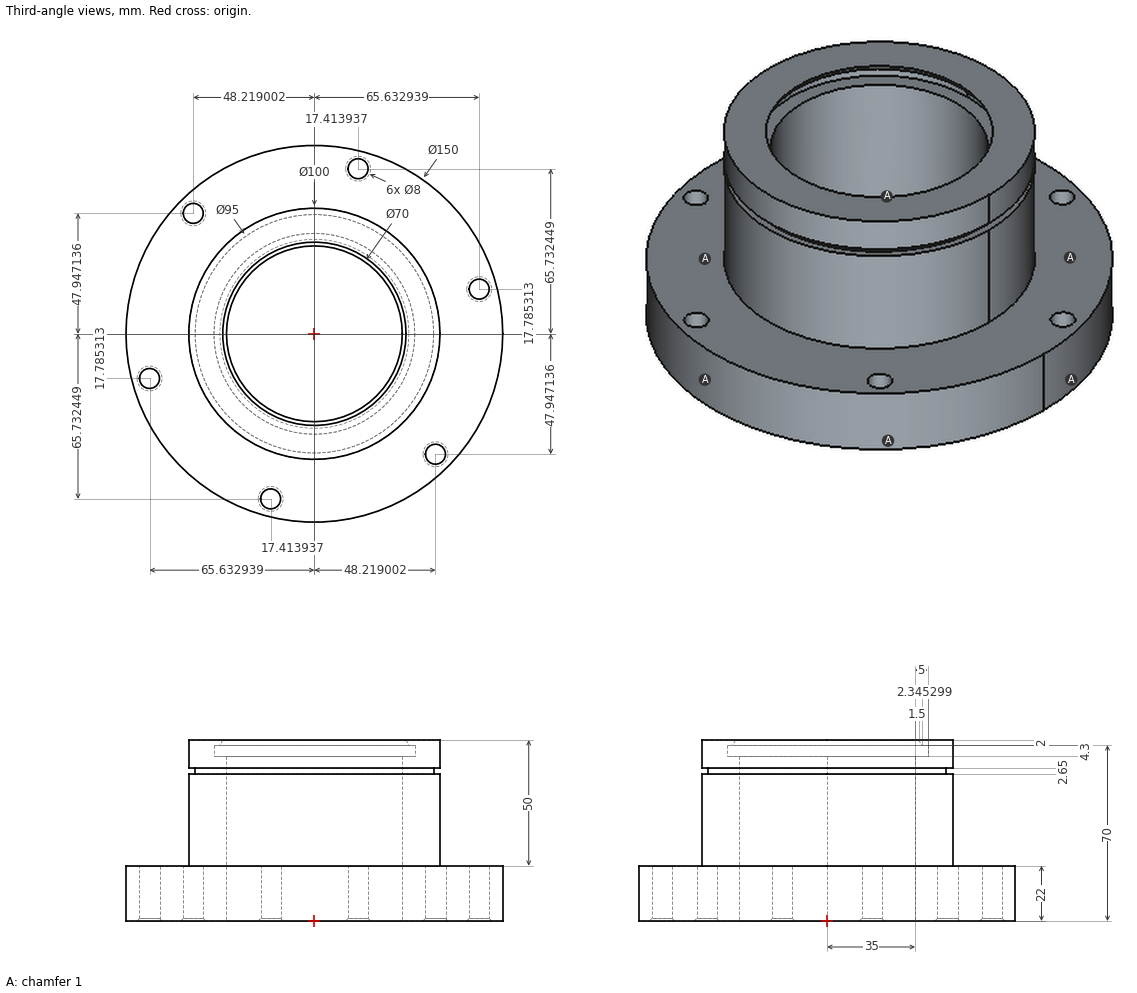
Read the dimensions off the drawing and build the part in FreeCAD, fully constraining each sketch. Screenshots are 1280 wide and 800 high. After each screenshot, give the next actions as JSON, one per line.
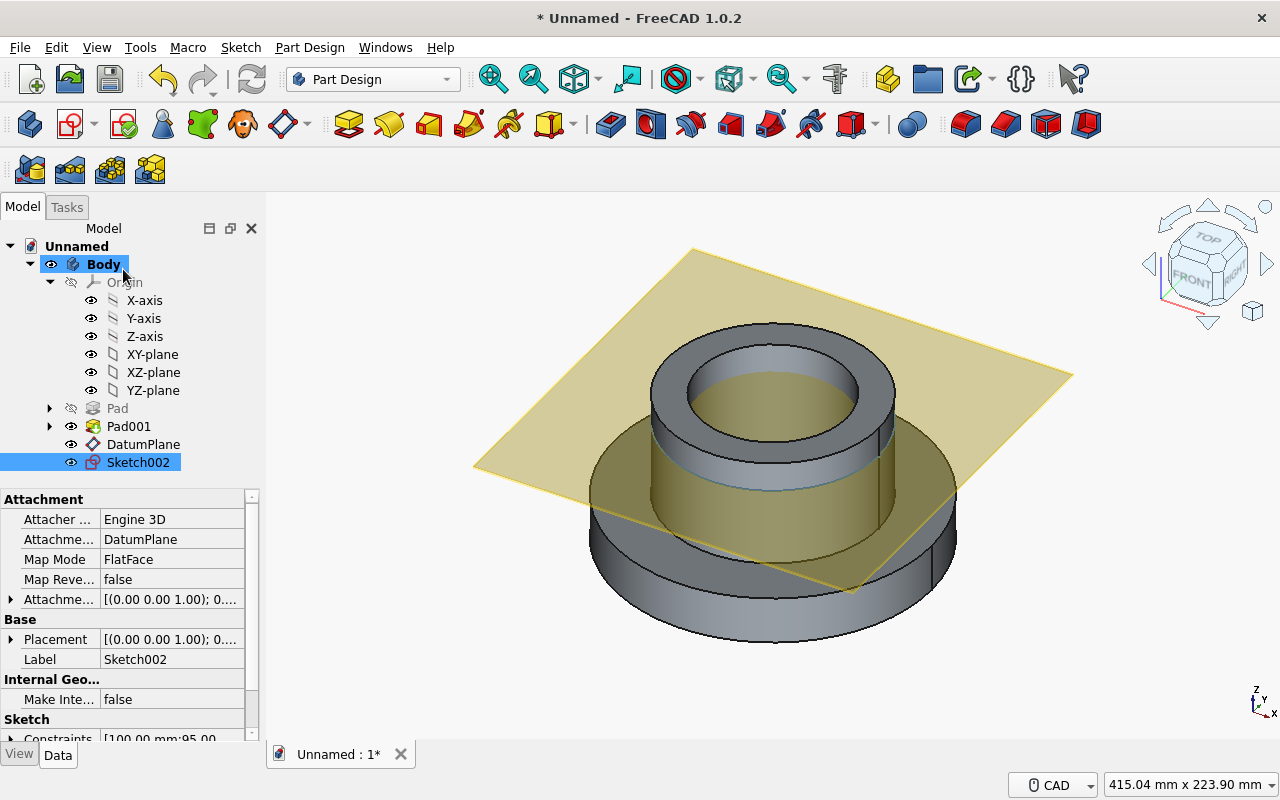
{"action": "left_click", "coordinate": [612, 124]}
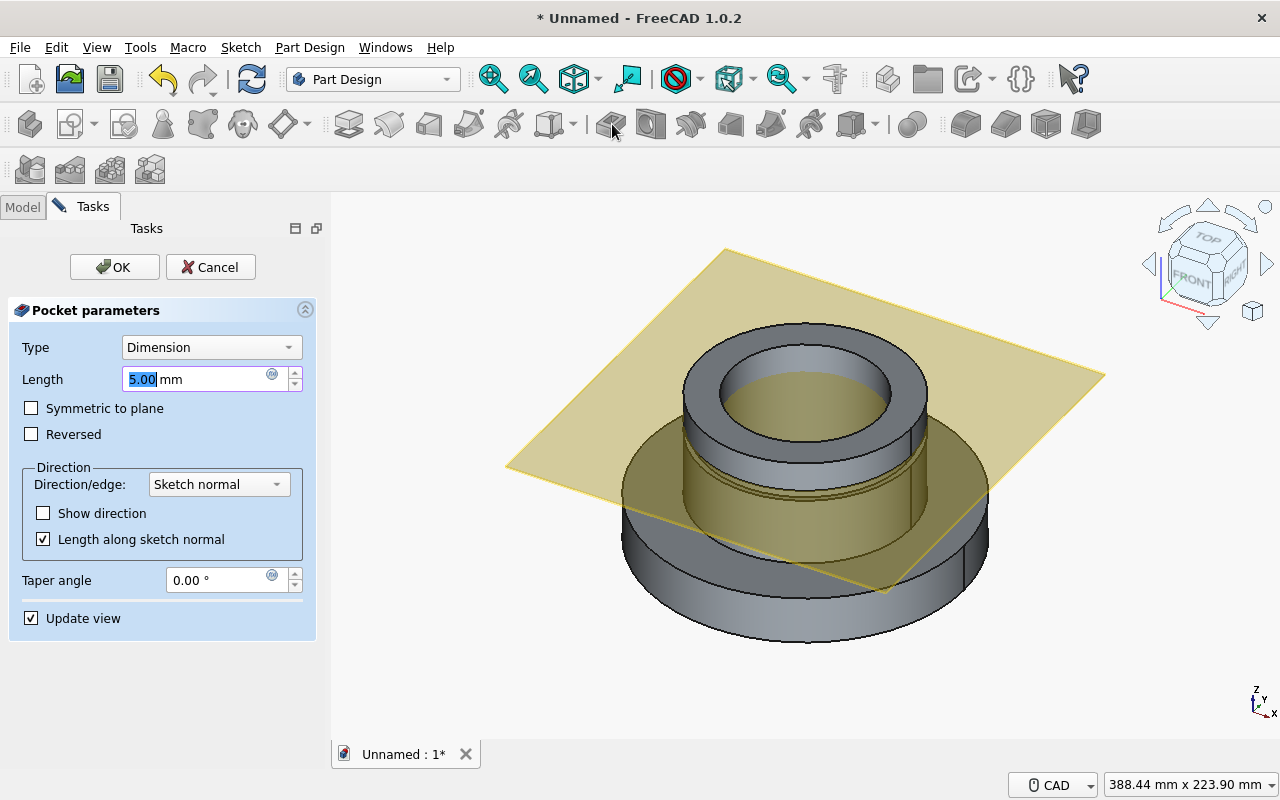
{"action": "type", "text": "2.65"}
{"action": "key", "text": "Tab"}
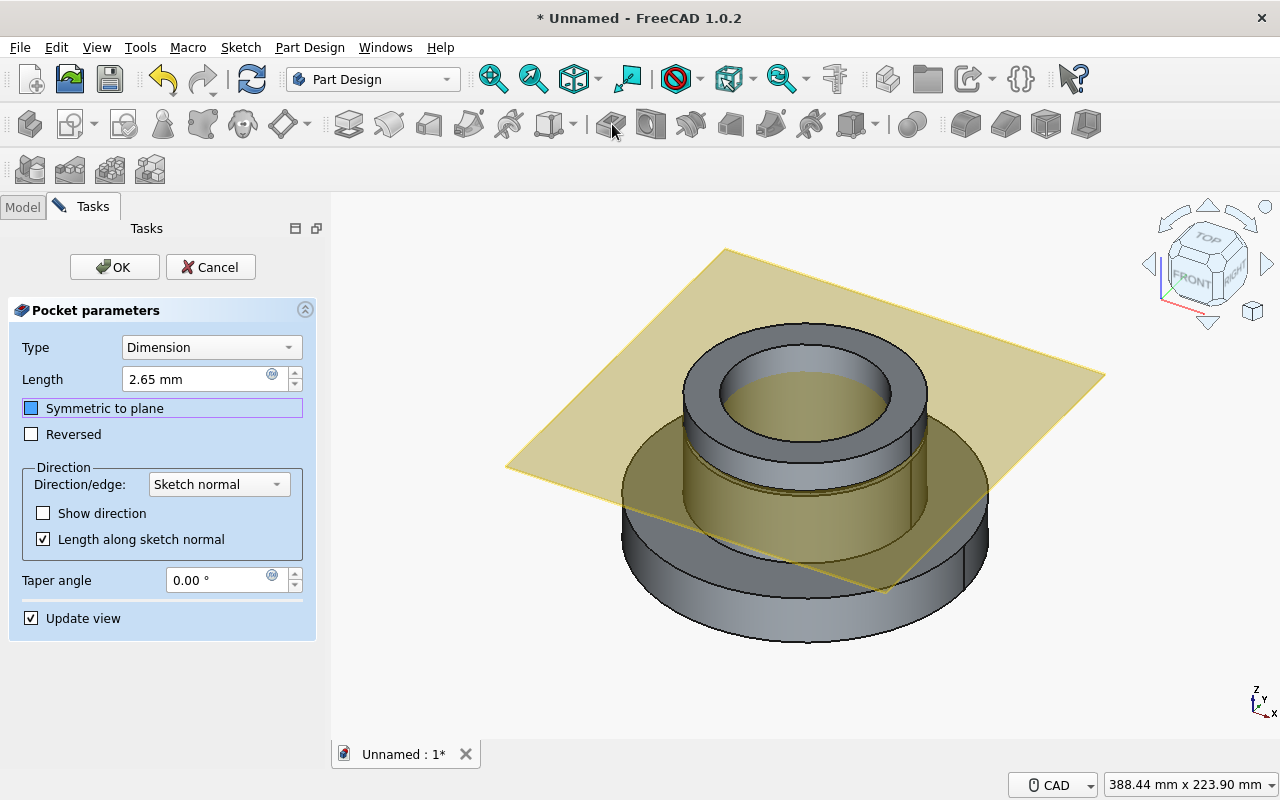
{"action": "left_click", "coordinate": [30, 434]}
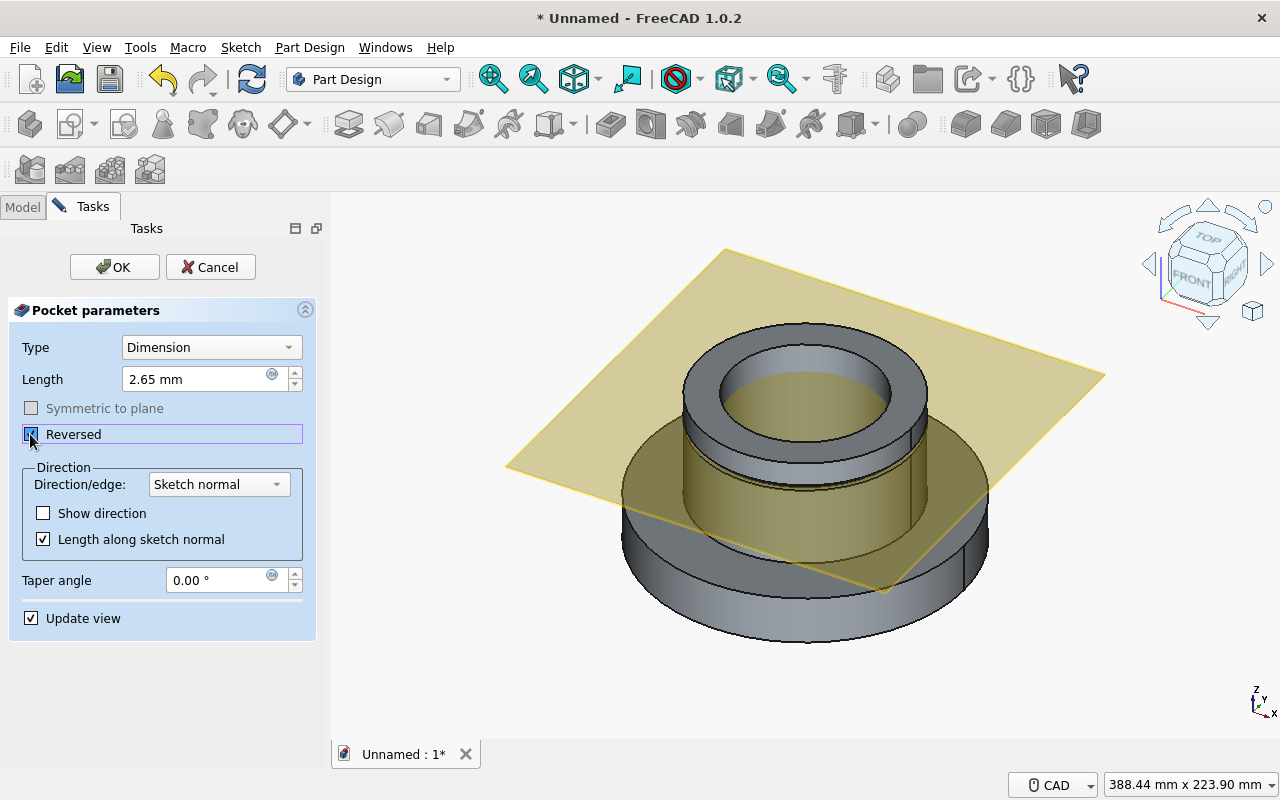
{"action": "left_click", "coordinate": [115, 267]}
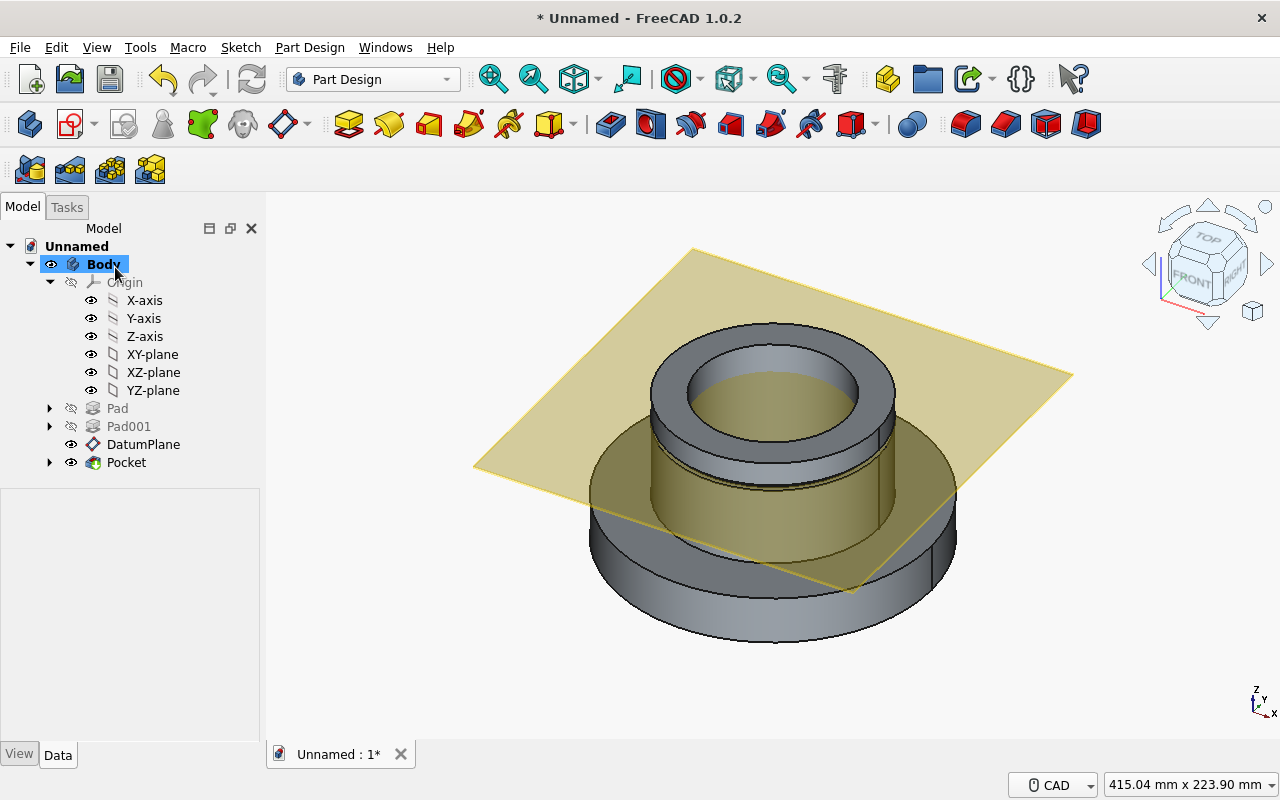
{"action": "left_click", "coordinate": [116, 444]}
{"action": "key", "text": "space"}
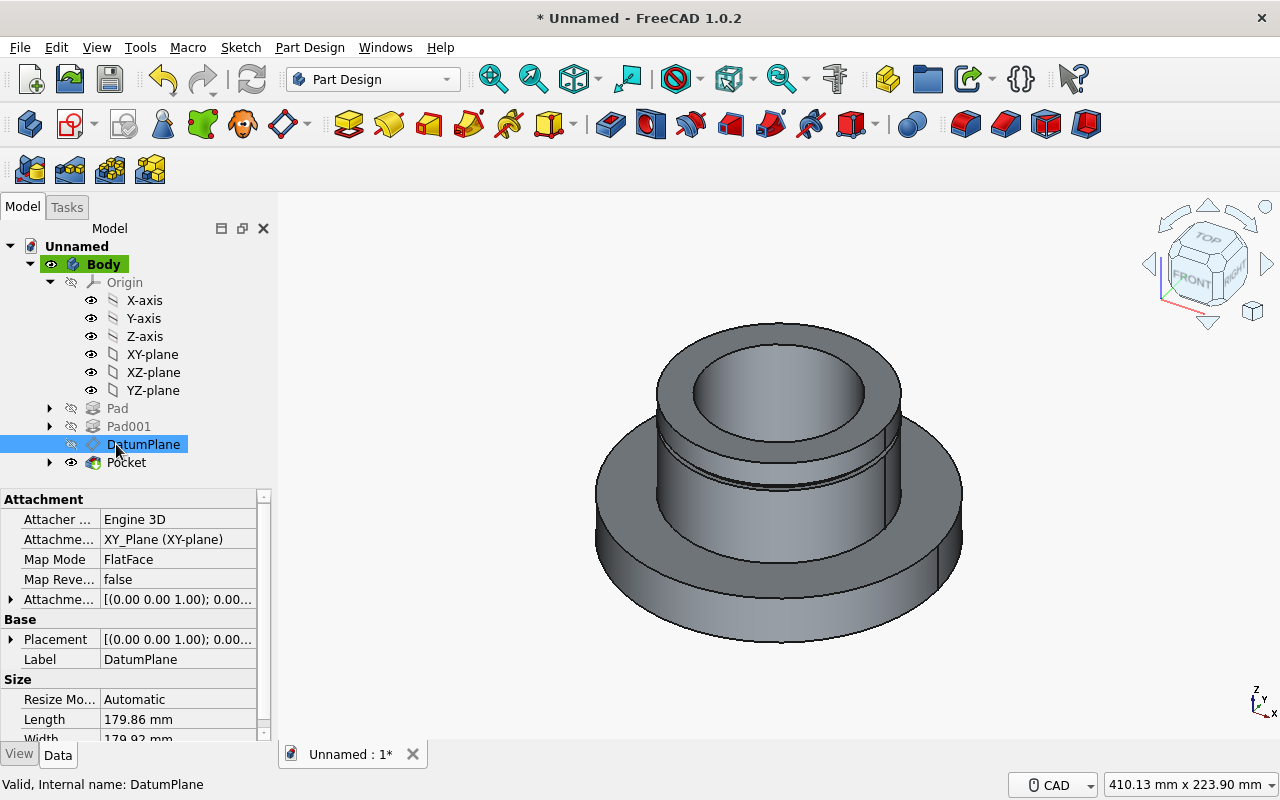
{"action": "left_click", "coordinate": [318, 699]}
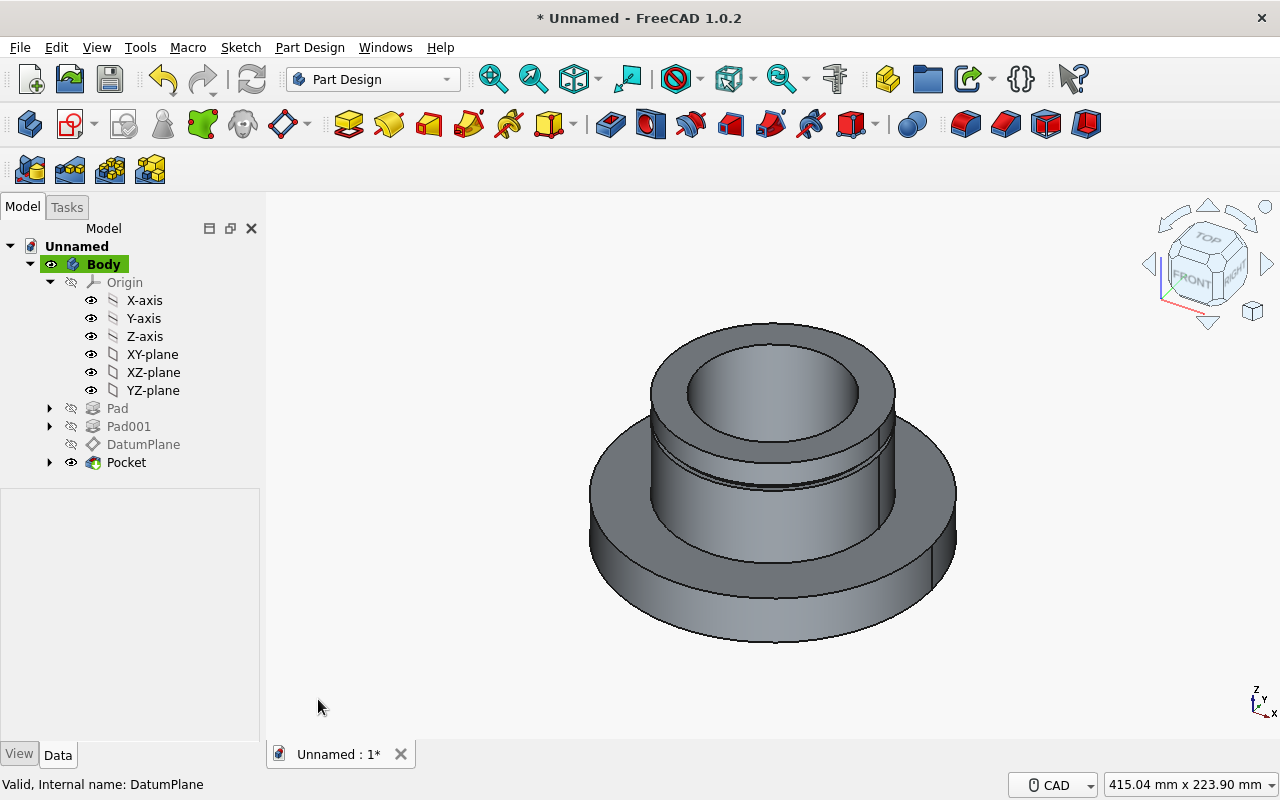
{"action": "left_click", "coordinate": [70, 124]}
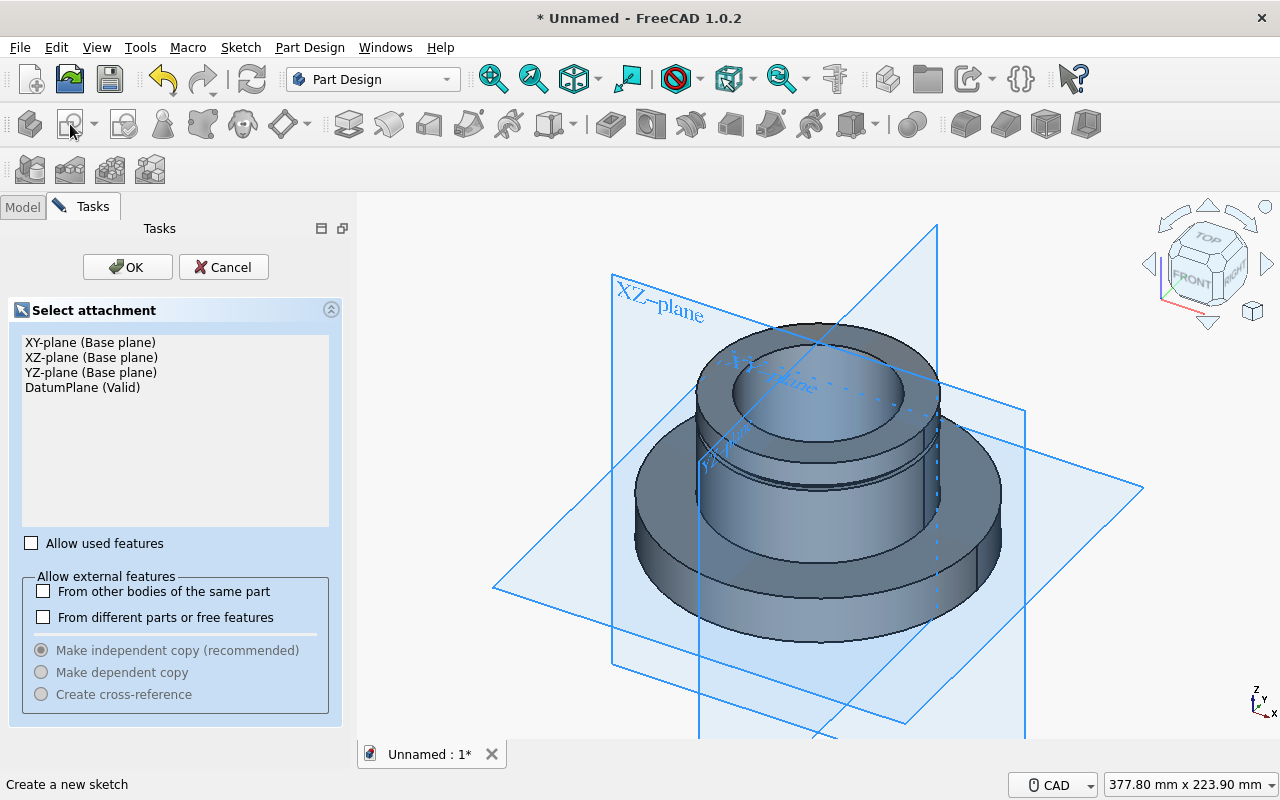
{"action": "left_click", "coordinate": [82, 342]}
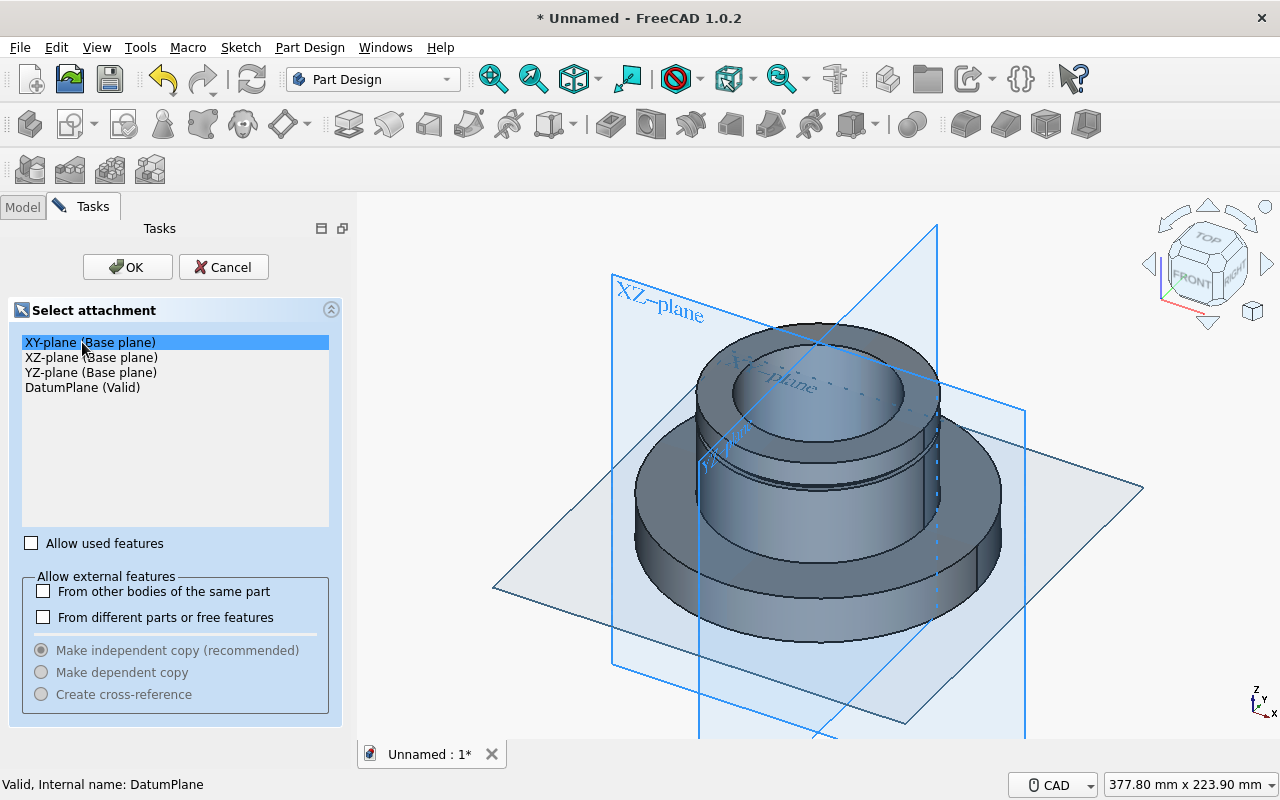
{"action": "left_click", "coordinate": [128, 267]}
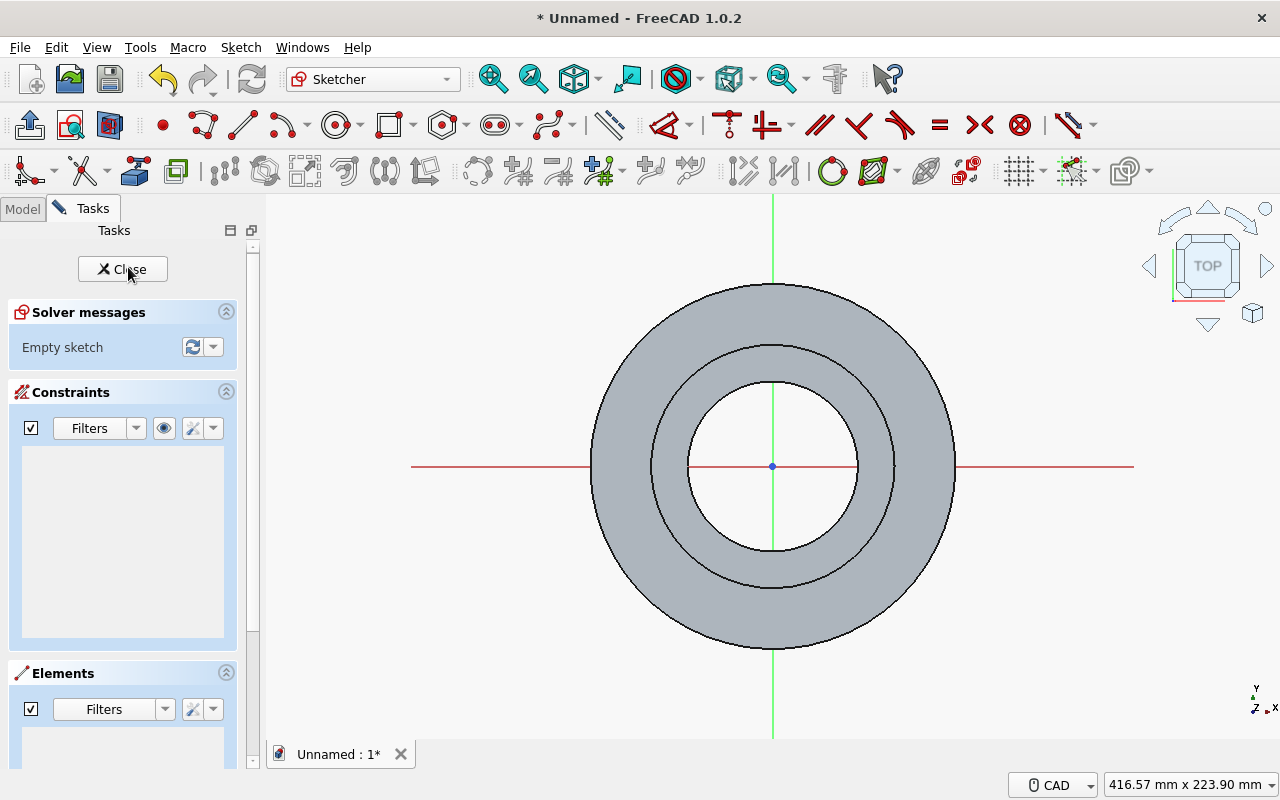
{"action": "left_click", "coordinate": [110, 126]}